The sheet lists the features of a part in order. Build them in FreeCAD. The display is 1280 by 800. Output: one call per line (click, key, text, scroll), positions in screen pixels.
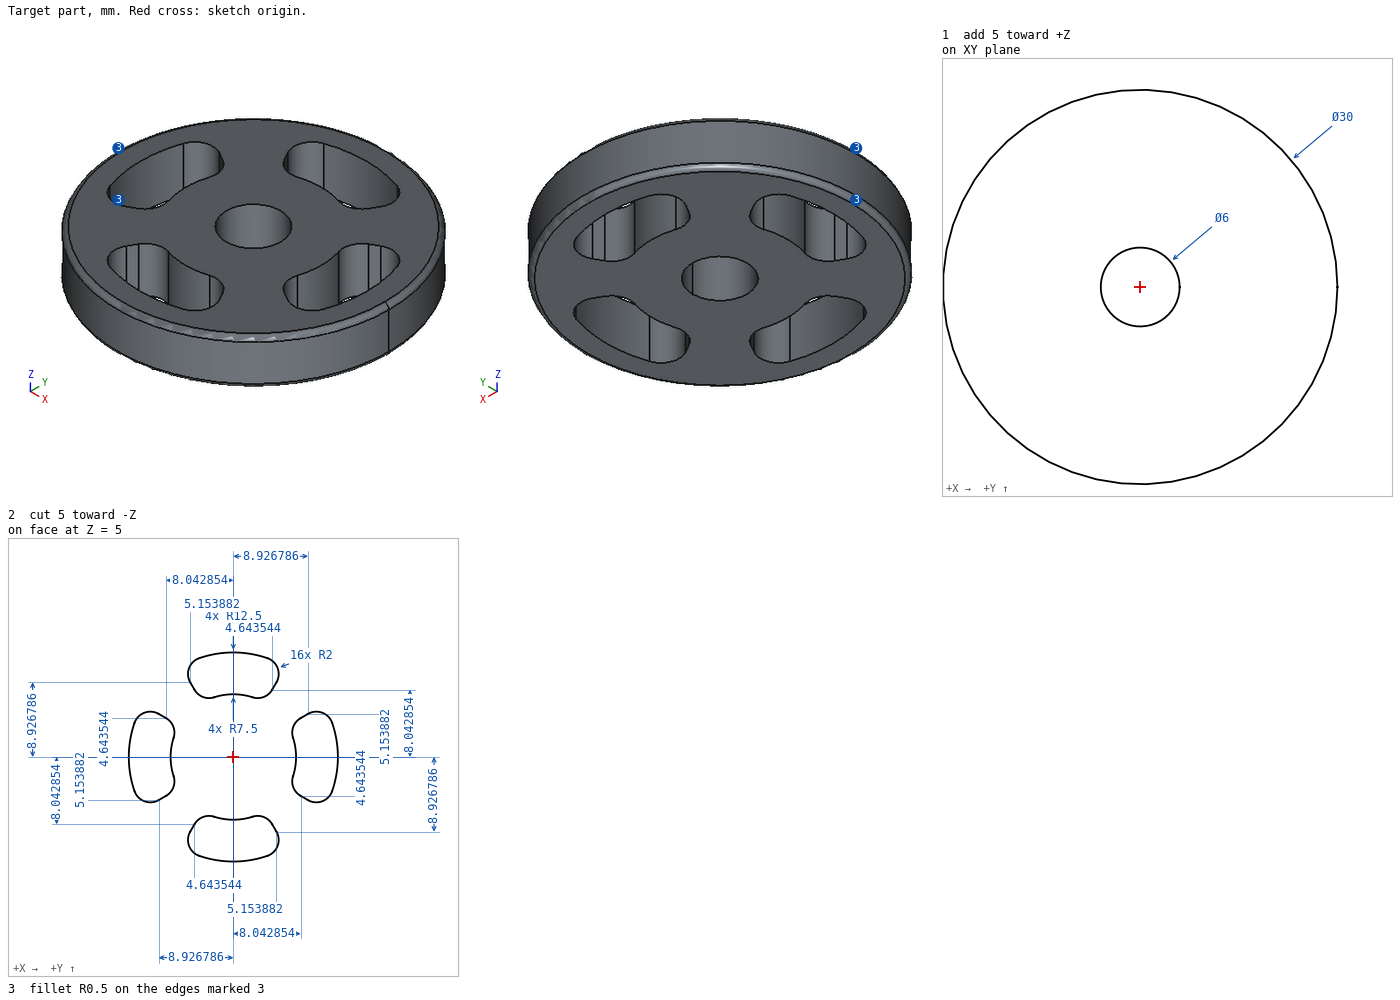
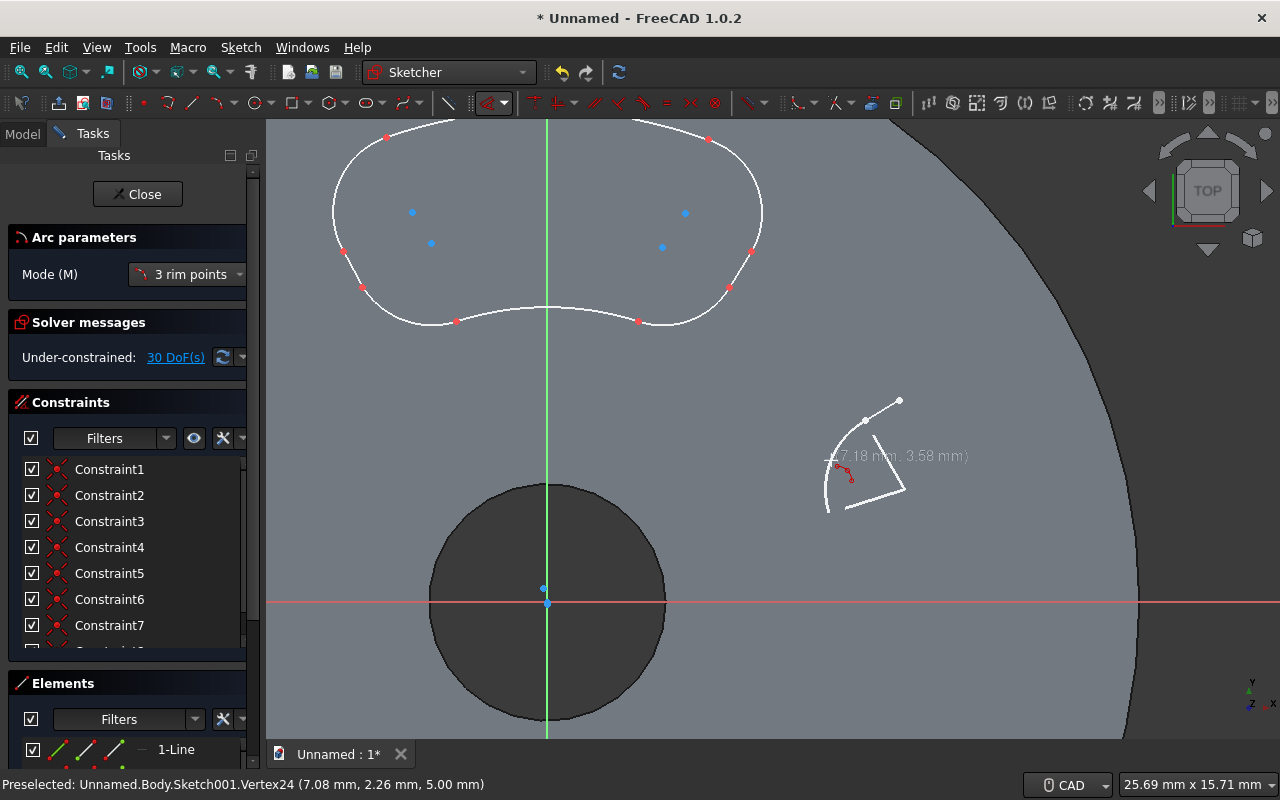
click(831, 459)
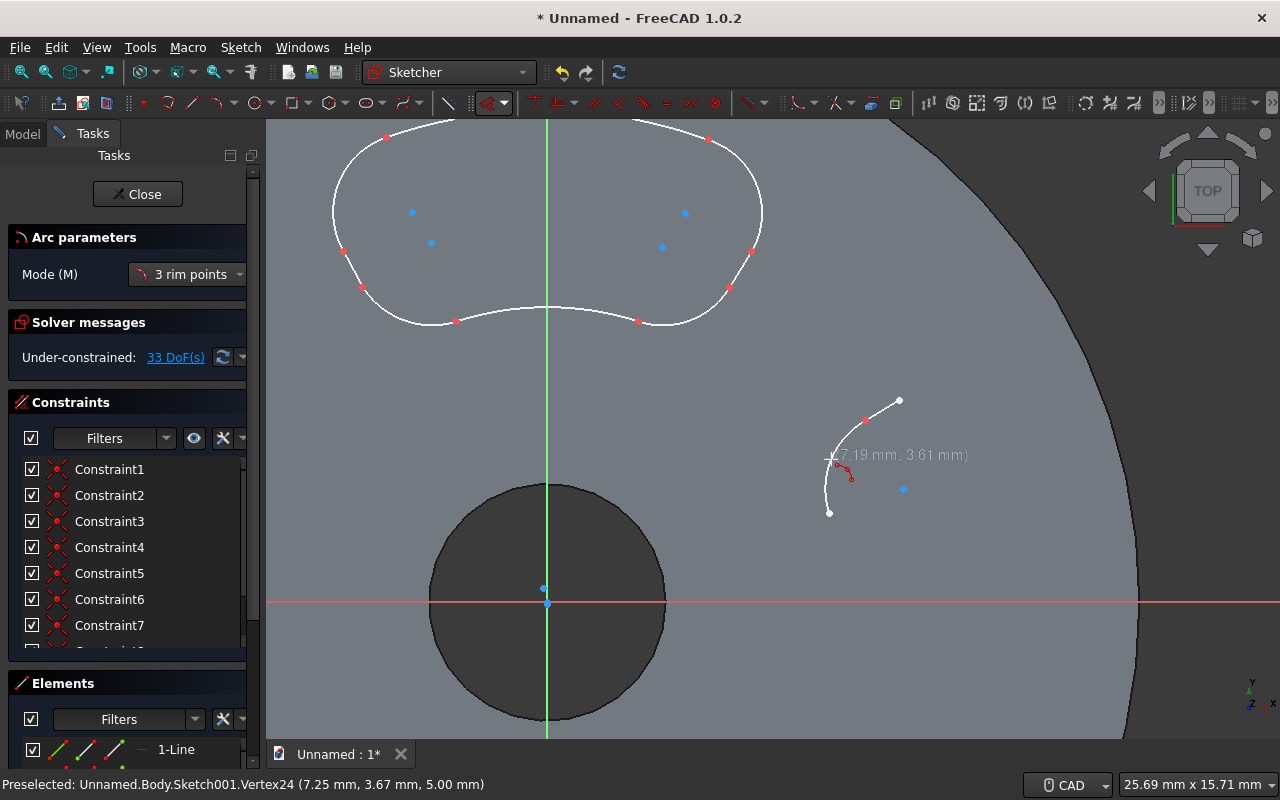
click(829, 513)
click(829, 693)
click(843, 621)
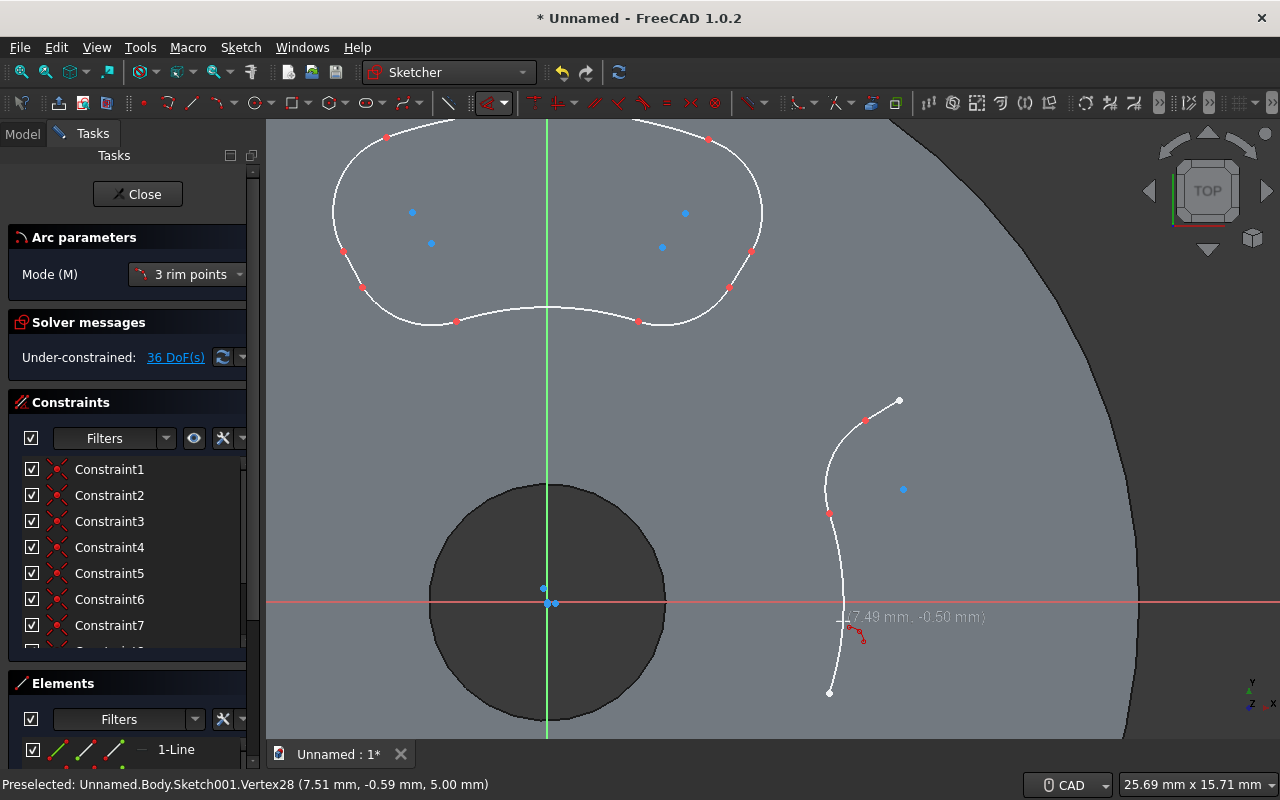
click(829, 694)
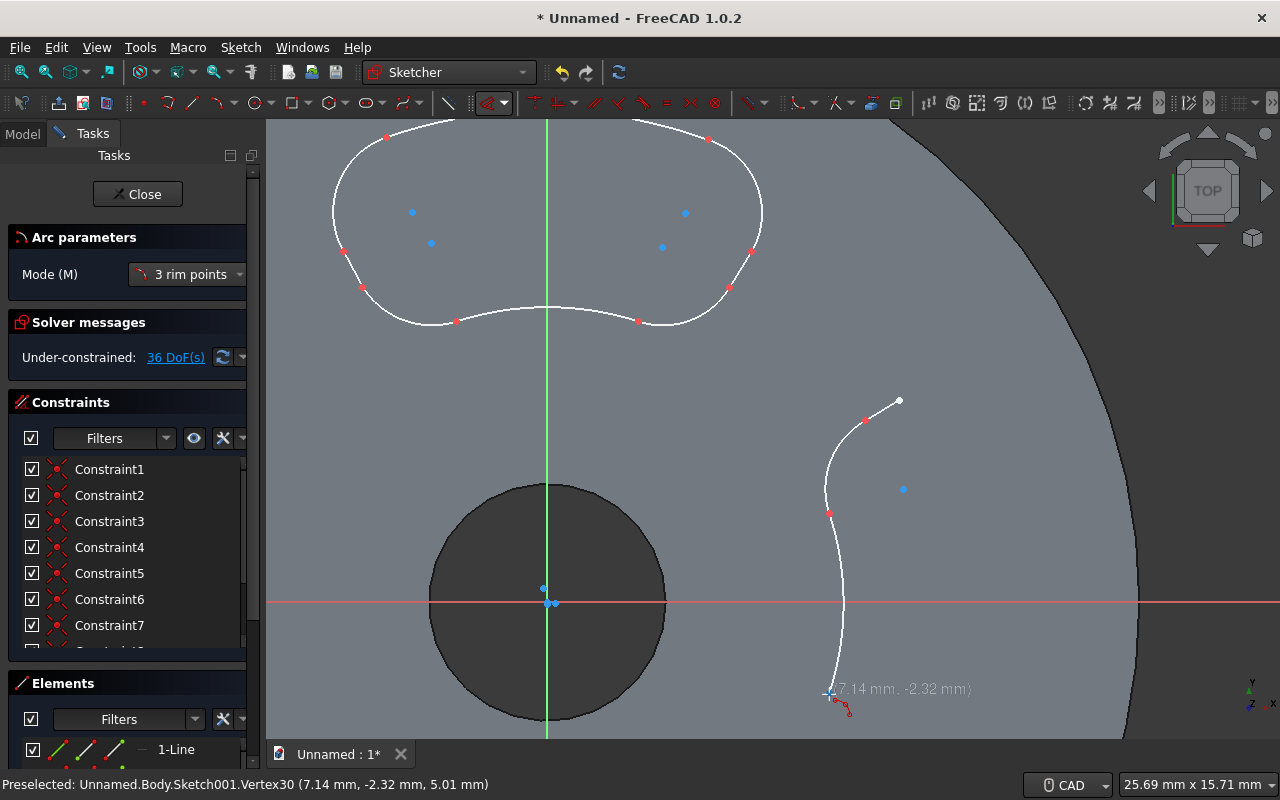
scroll(796, 328, down, 5)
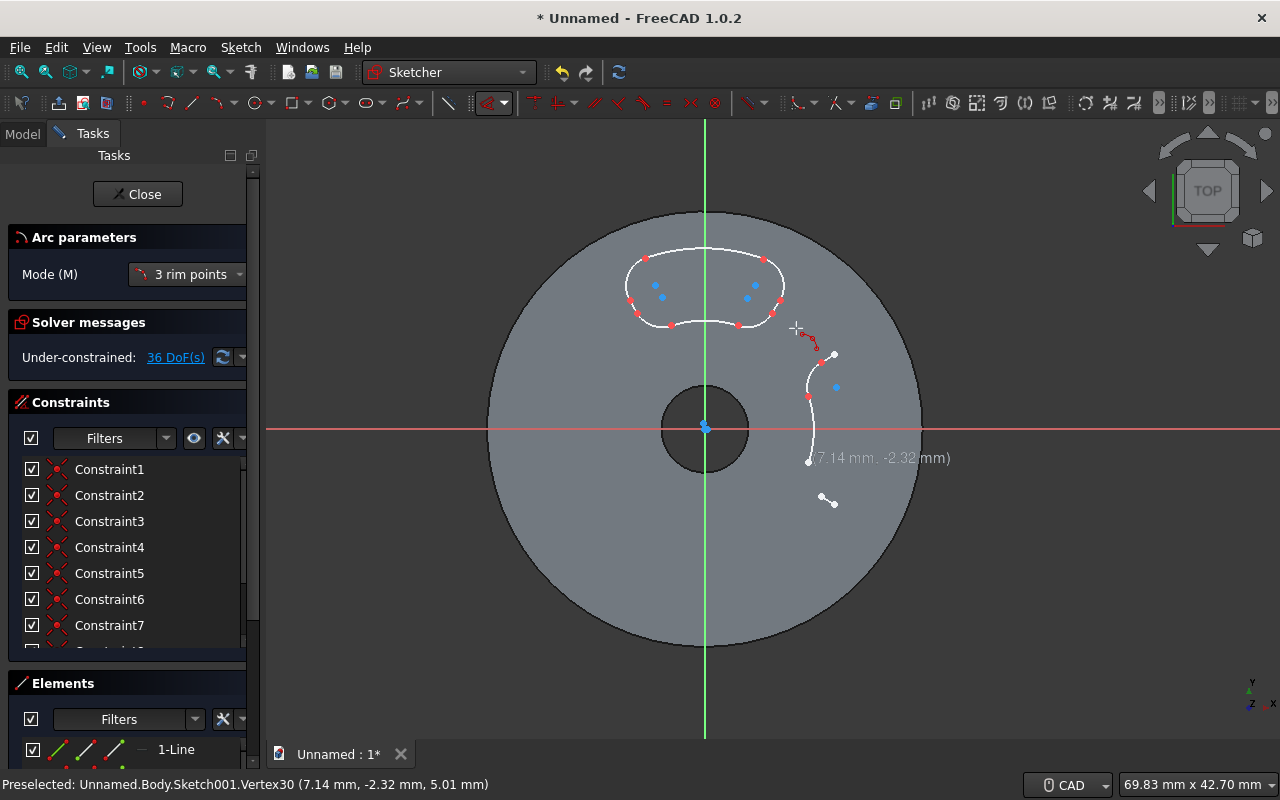
scroll(822, 497, up, 4)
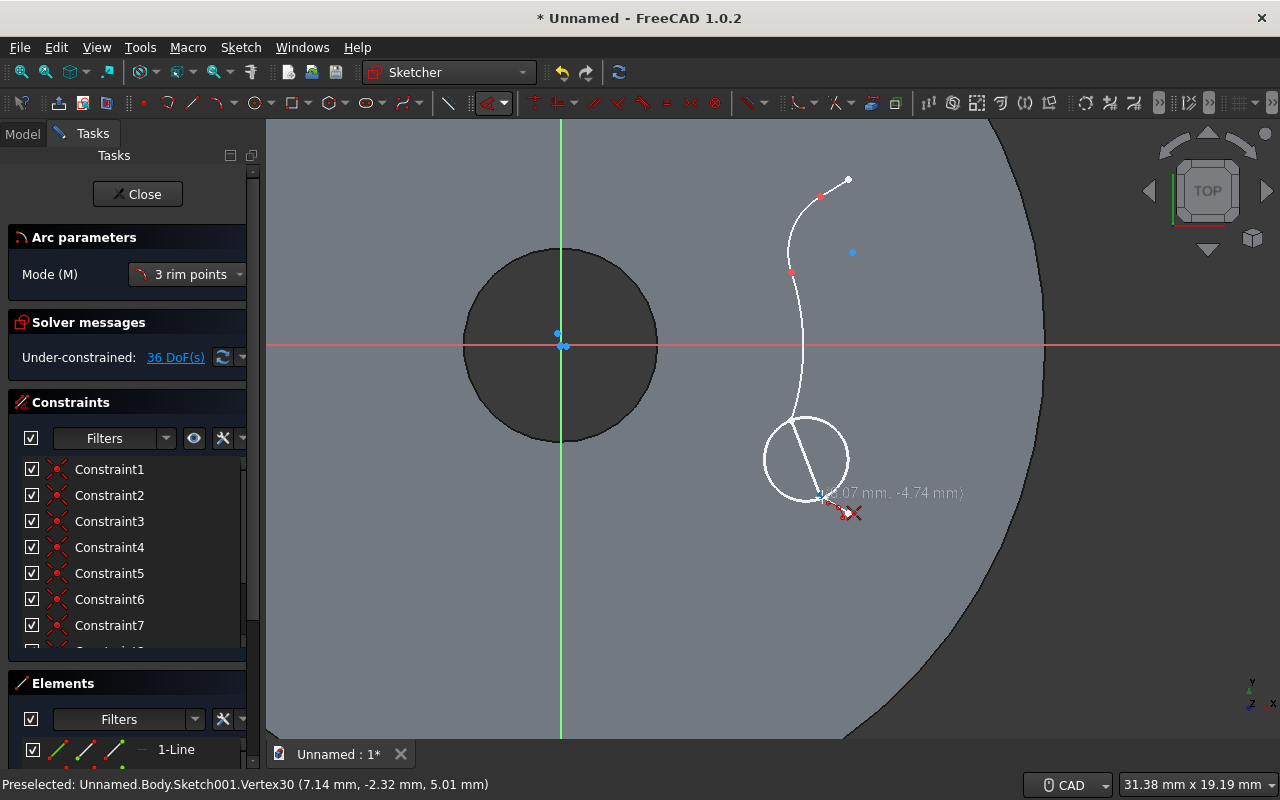
click(821, 496)
click(793, 463)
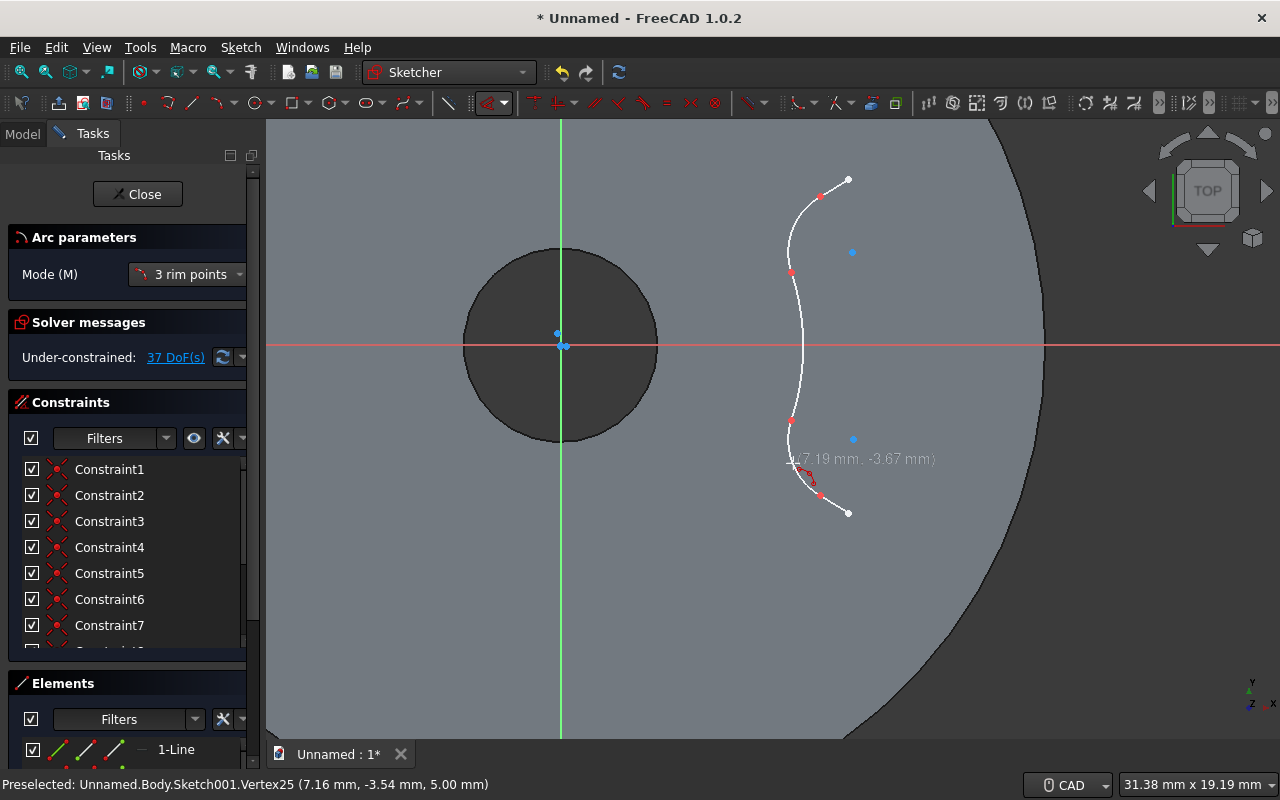
click(849, 513)
click(942, 477)
click(904, 516)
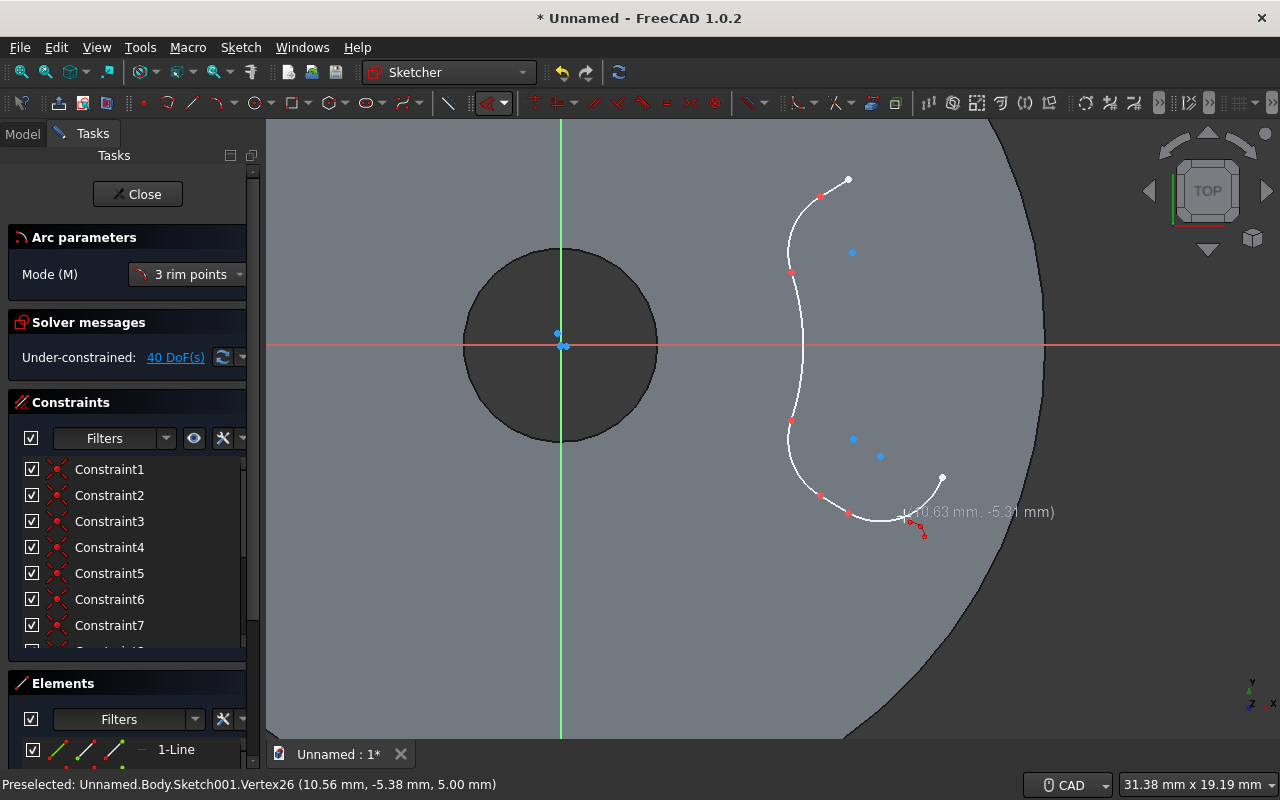
click(942, 478)
click(942, 214)
click(964, 372)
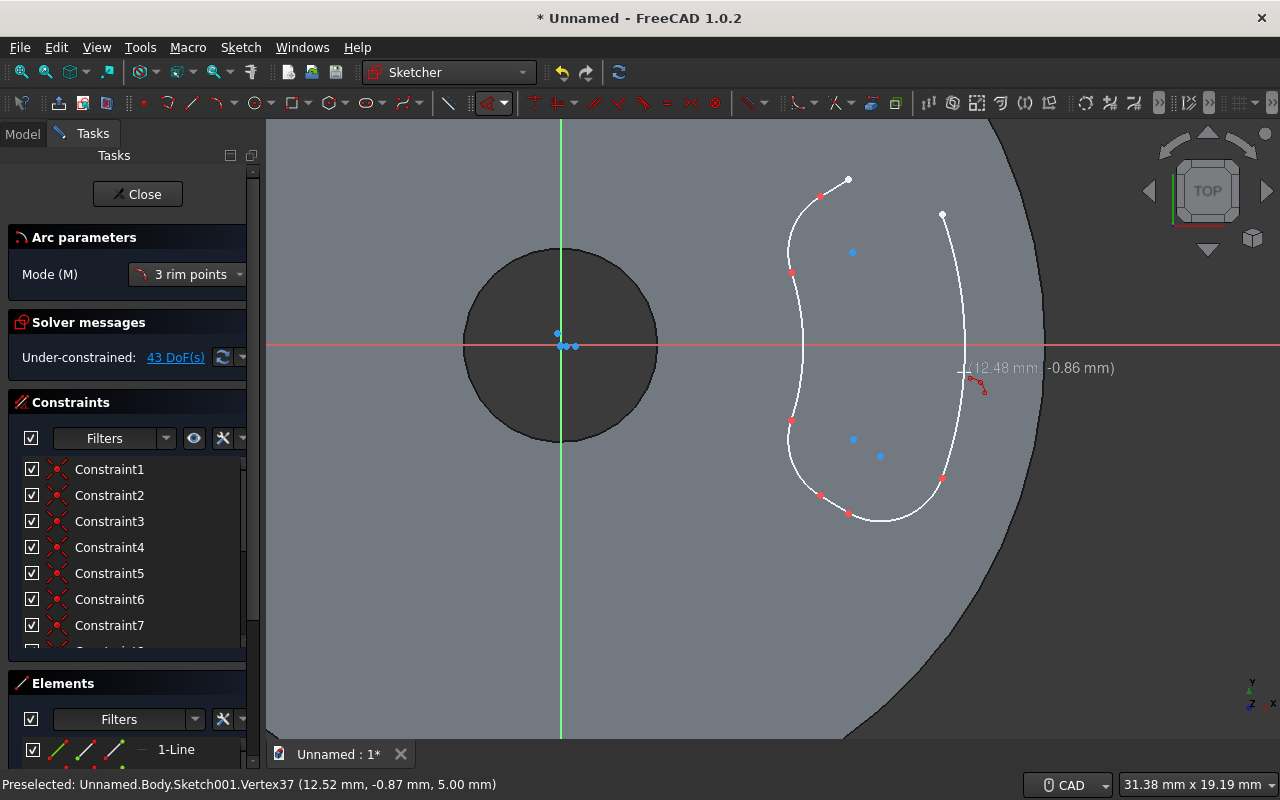
click(942, 215)
click(849, 180)
click(904, 174)